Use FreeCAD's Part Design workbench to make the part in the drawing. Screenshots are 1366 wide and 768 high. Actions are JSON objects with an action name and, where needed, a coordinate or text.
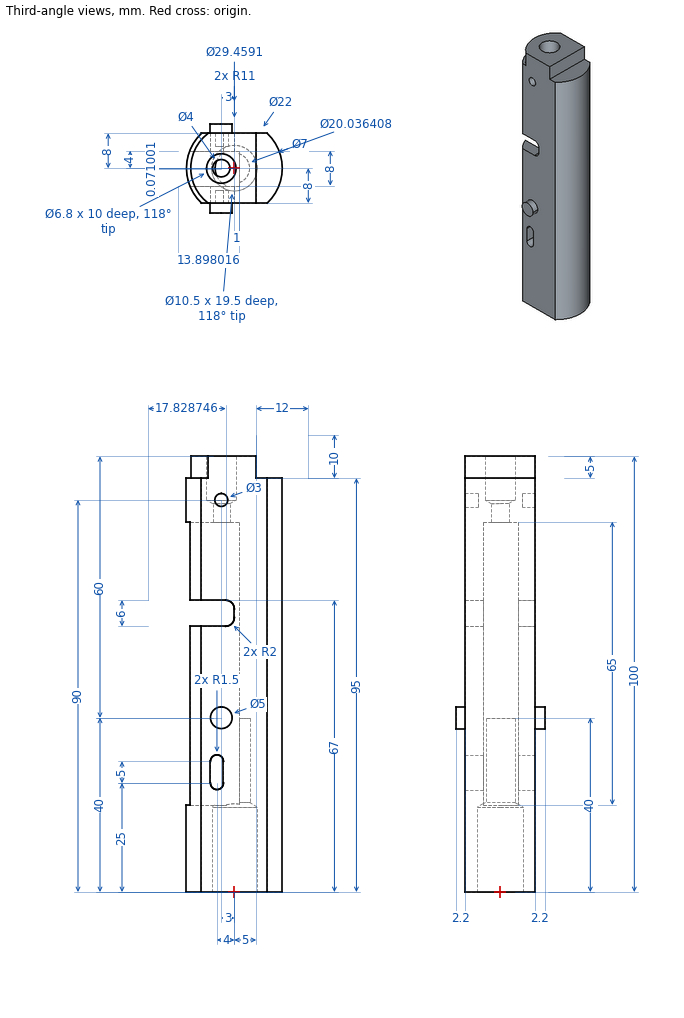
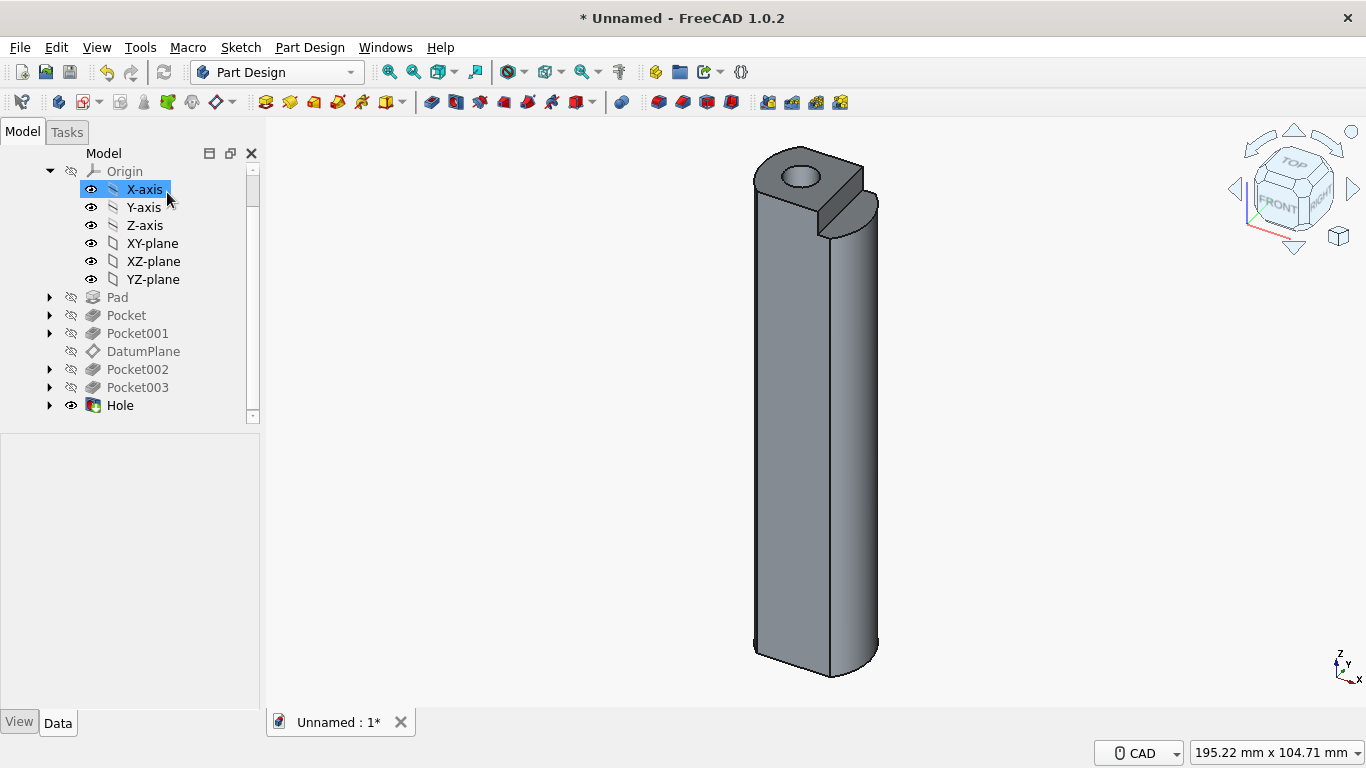
{"action": "left_click", "coordinate": [136, 261]}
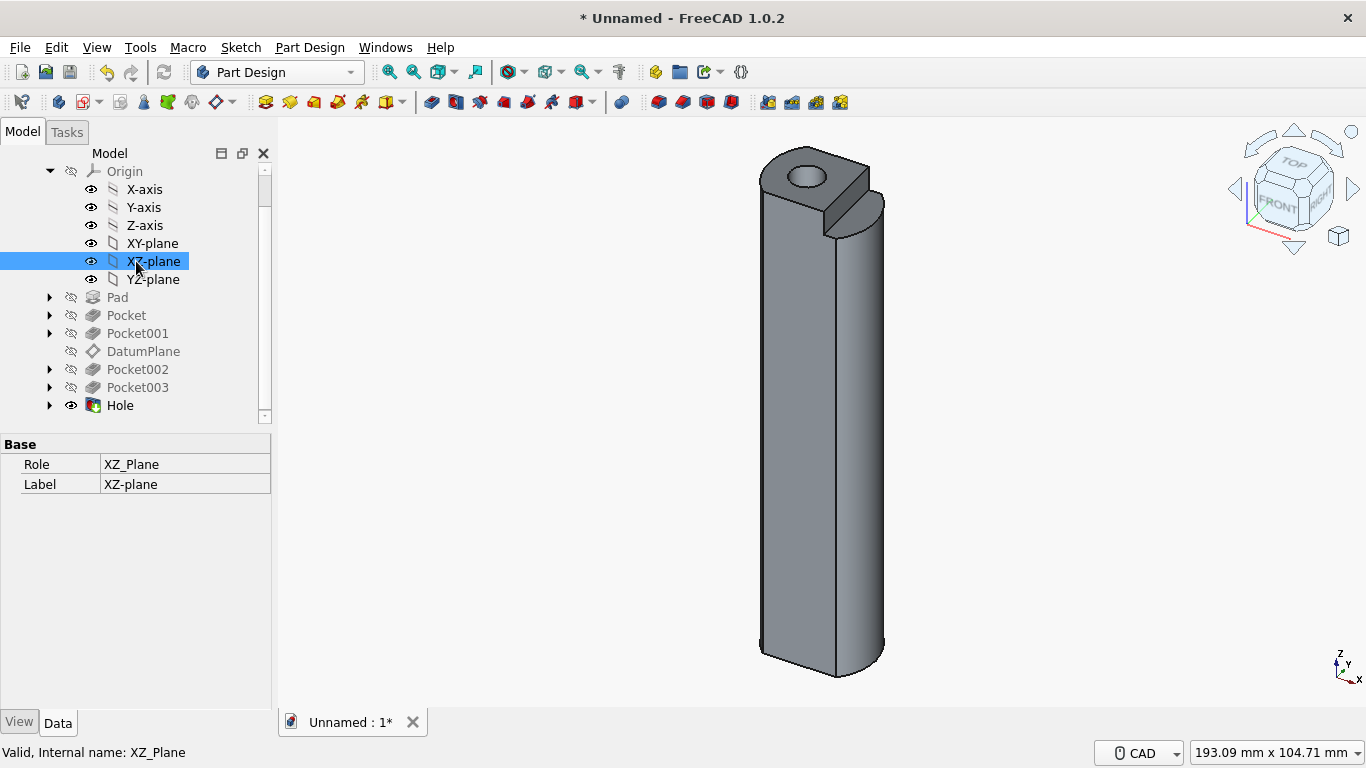
{"action": "left_click", "coordinate": [216, 102]}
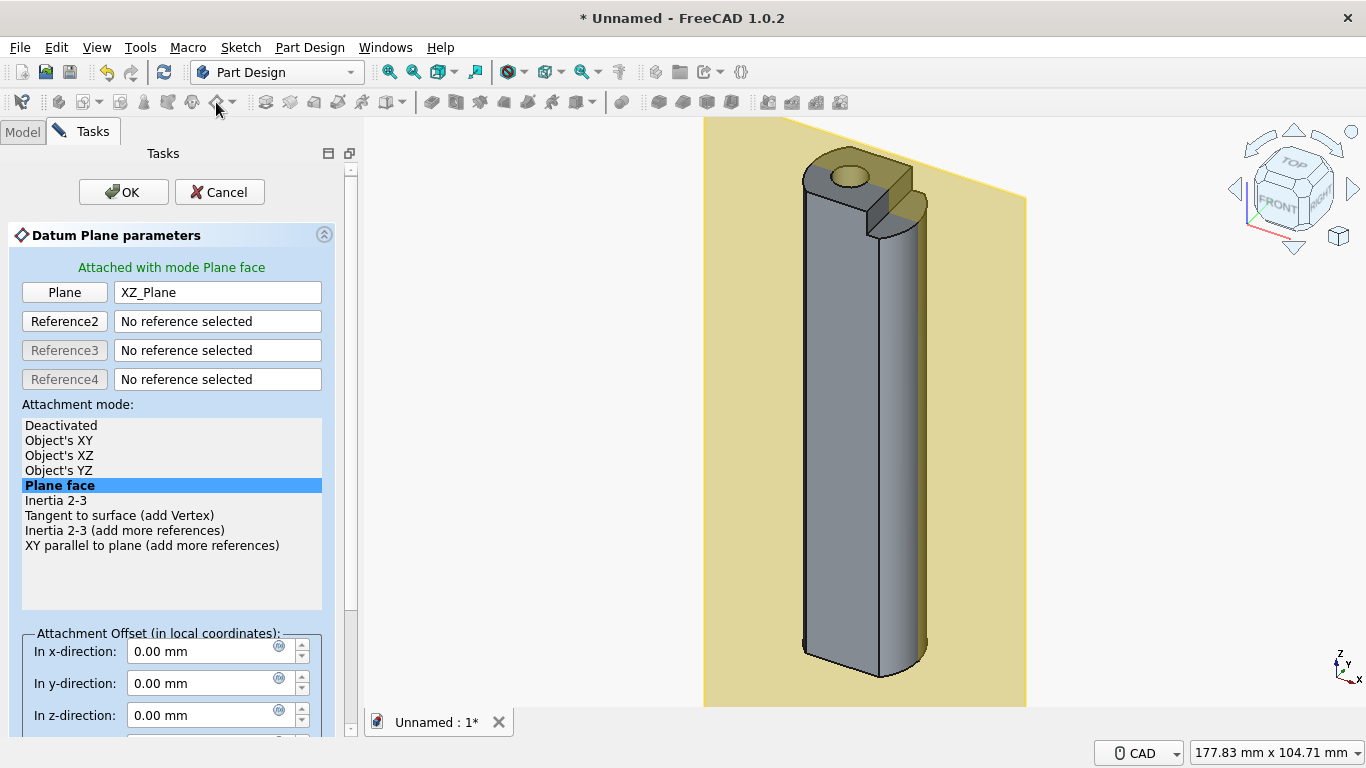
{"action": "triple_click", "coordinate": [210, 715]}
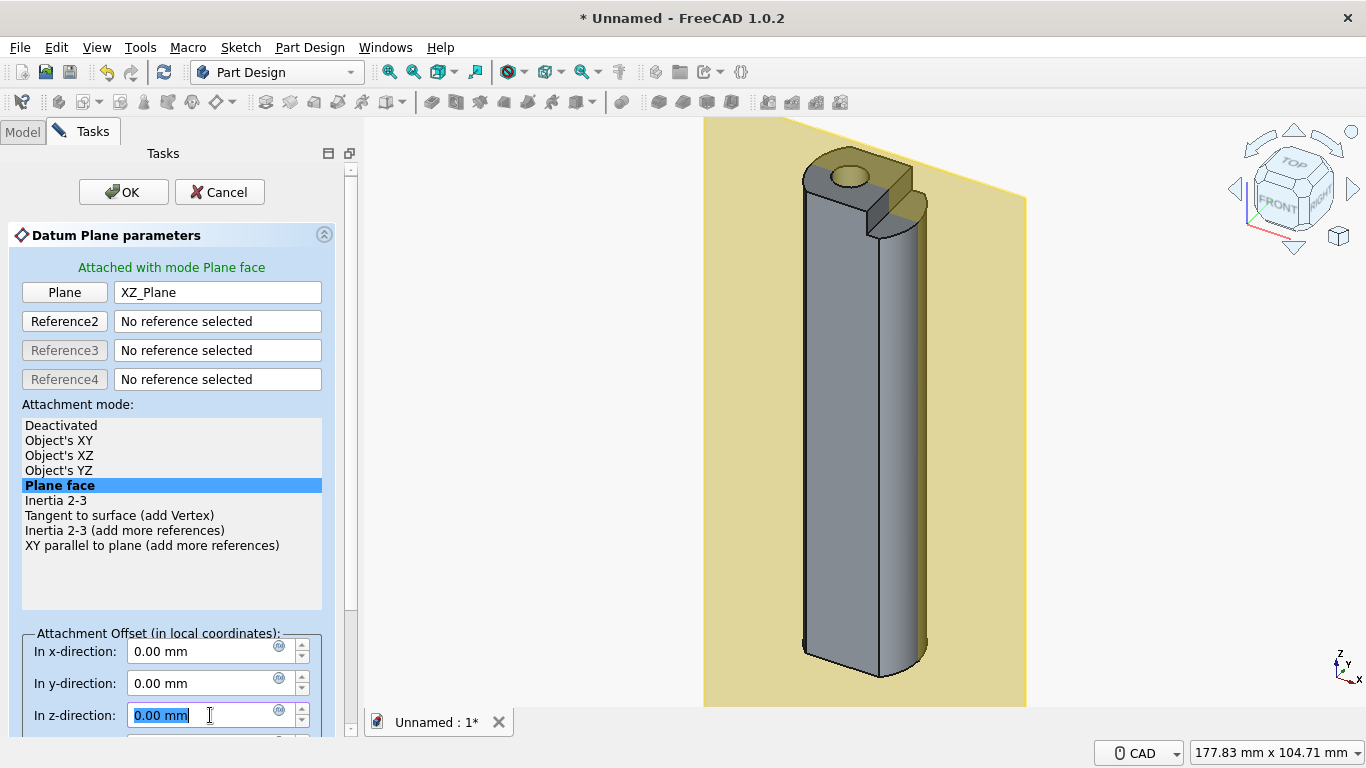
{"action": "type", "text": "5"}
{"action": "key", "text": "Tab"}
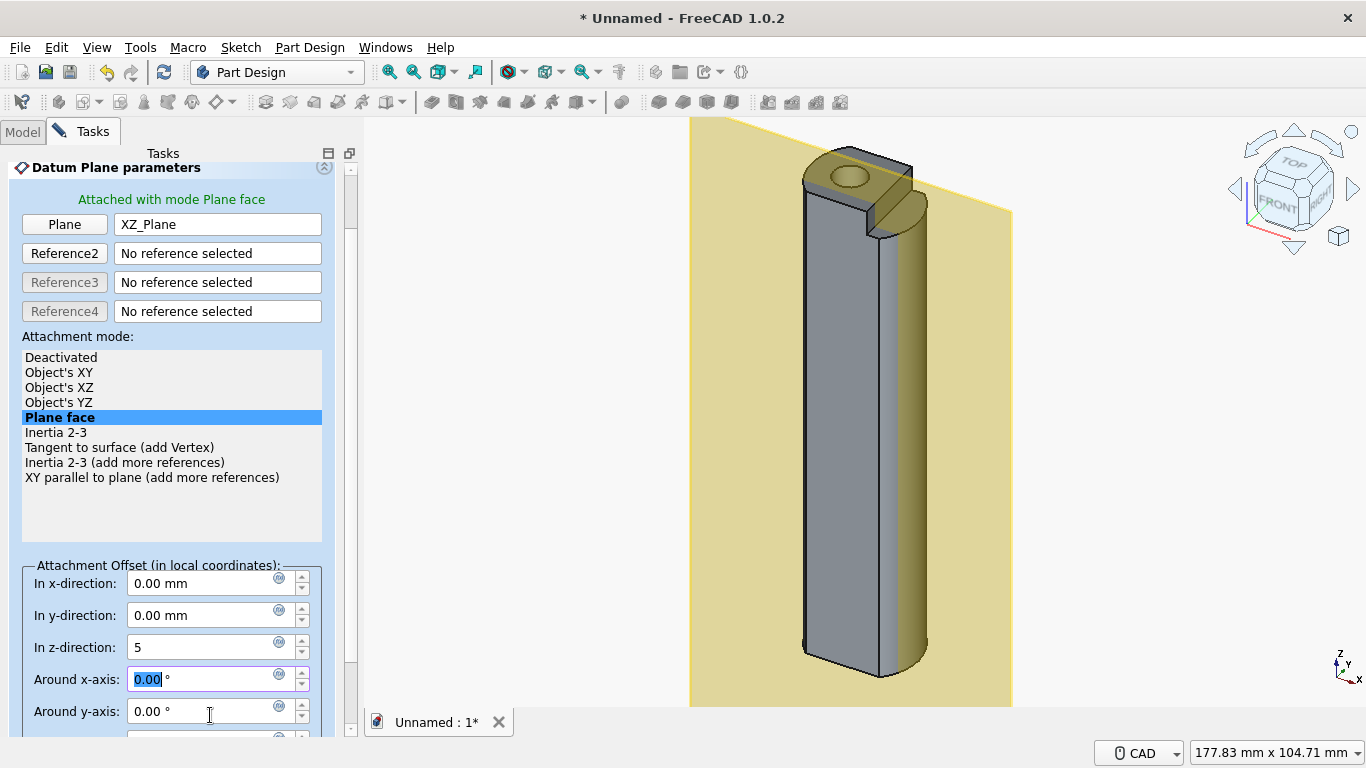
{"action": "scroll", "coordinate": [351, 450], "scroll_direction": "up", "scroll_amount": 2}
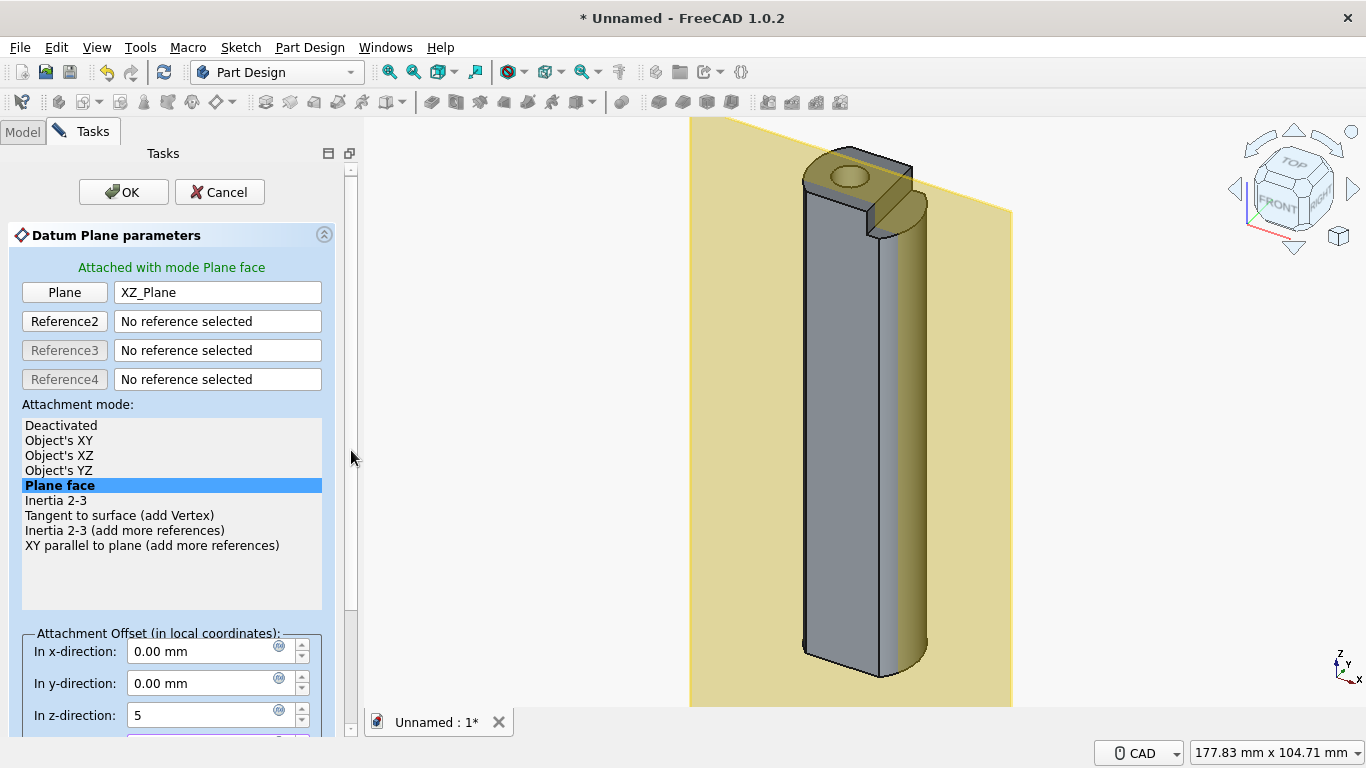
{"action": "left_click", "coordinate": [124, 192]}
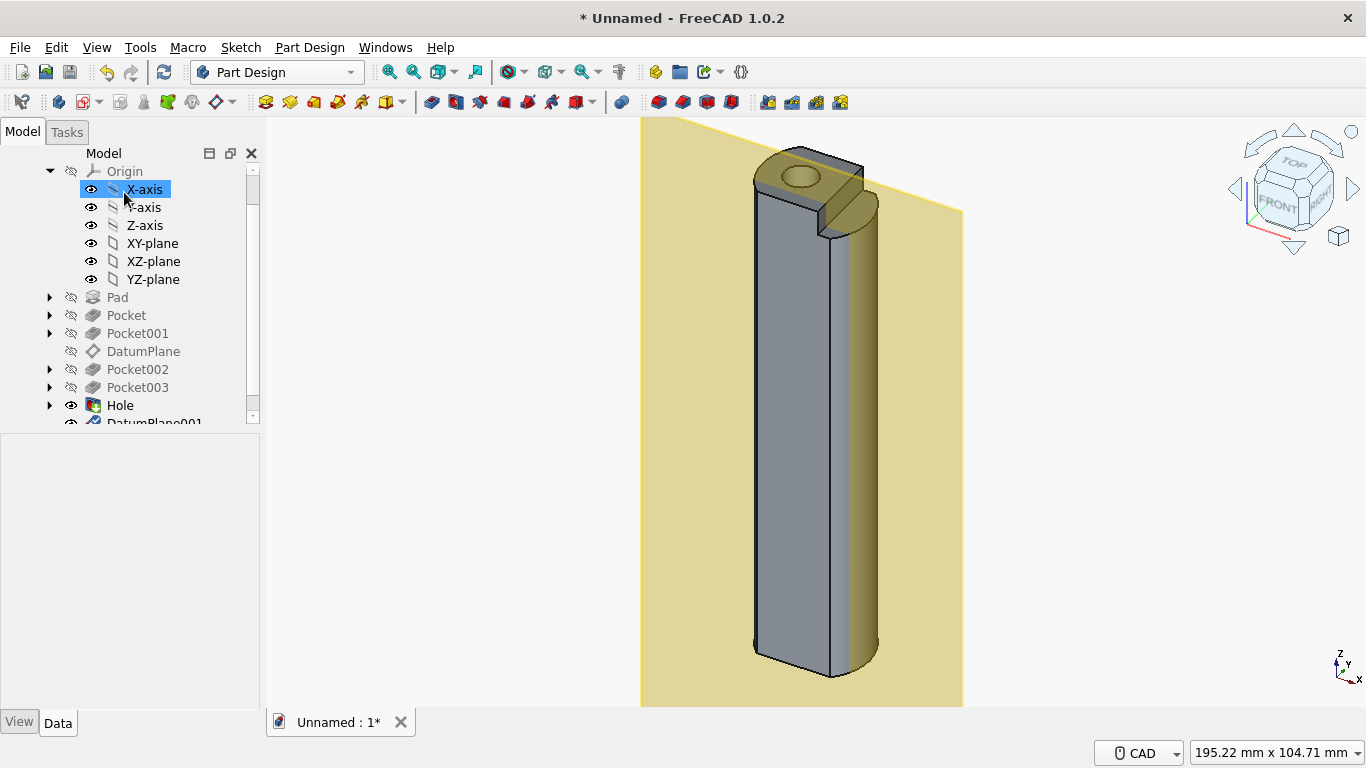
{"action": "left_click", "coordinate": [116, 423]}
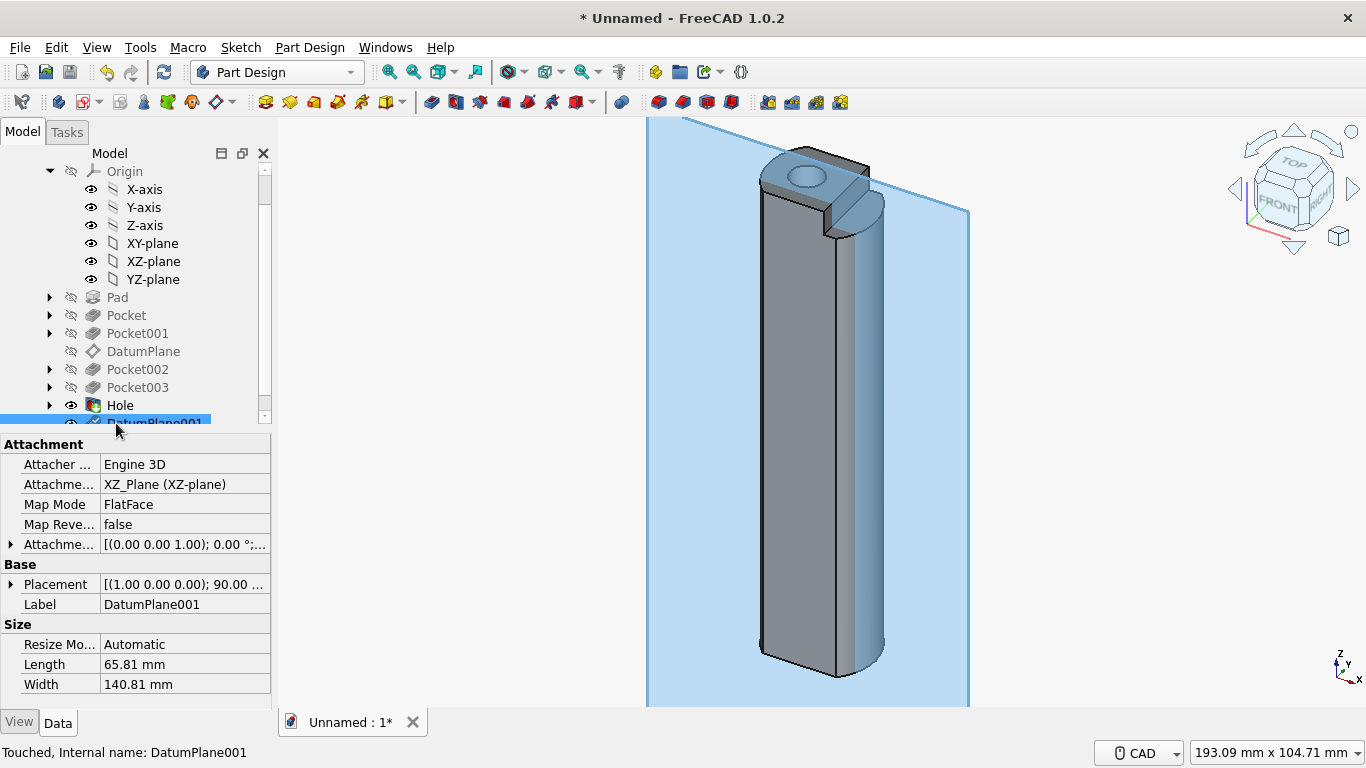
{"action": "left_click", "coordinate": [84, 102]}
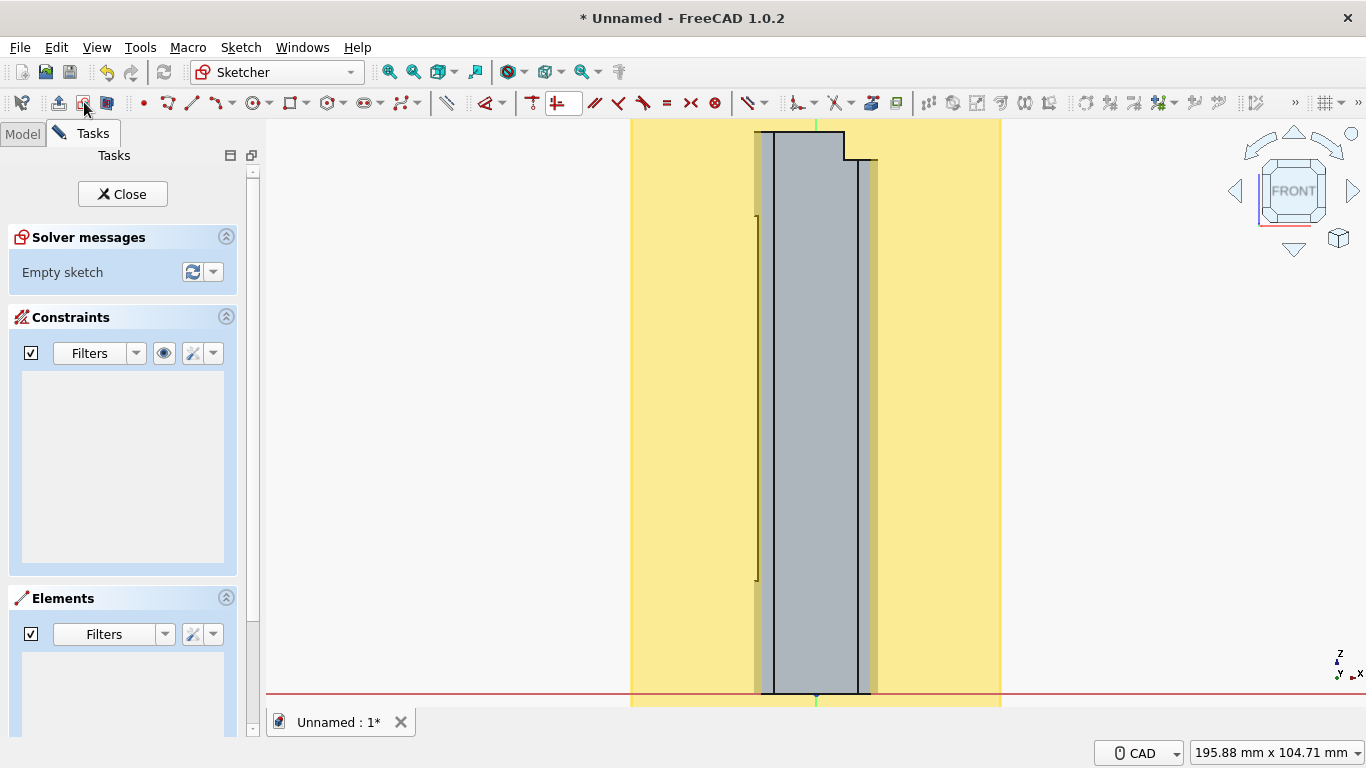
{"action": "left_click", "coordinate": [108, 104]}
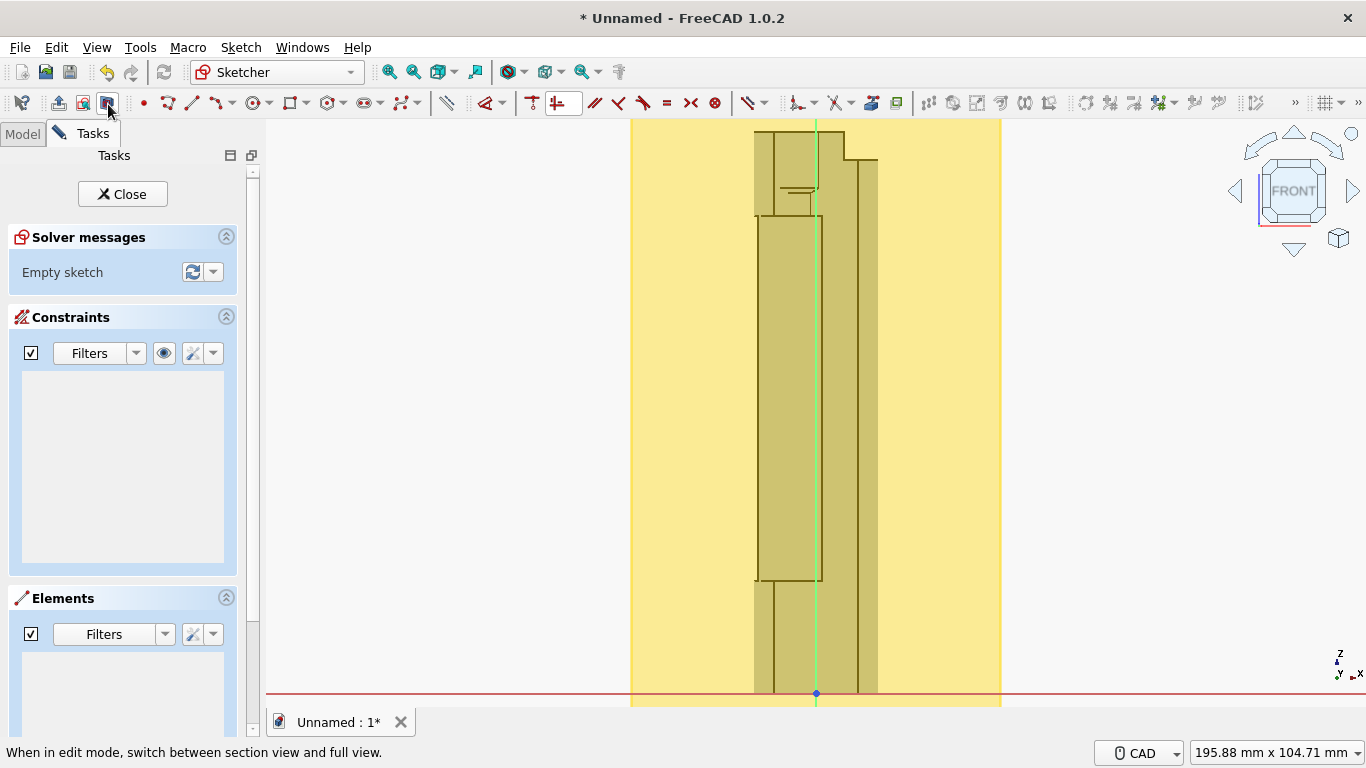
{"action": "scroll", "coordinate": [802, 177], "scroll_direction": "up", "scroll_amount": 15}